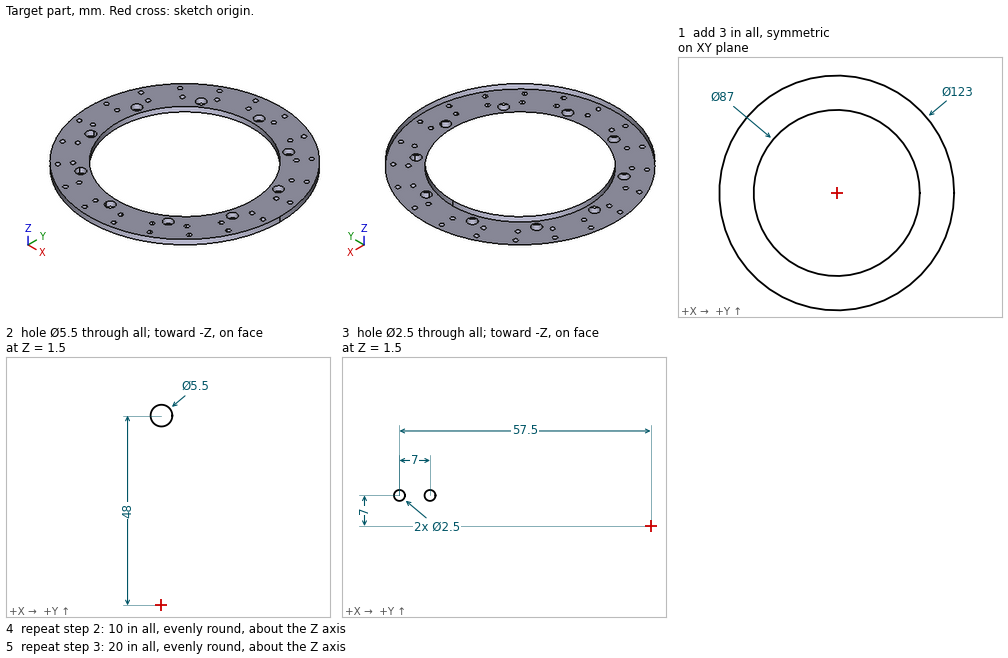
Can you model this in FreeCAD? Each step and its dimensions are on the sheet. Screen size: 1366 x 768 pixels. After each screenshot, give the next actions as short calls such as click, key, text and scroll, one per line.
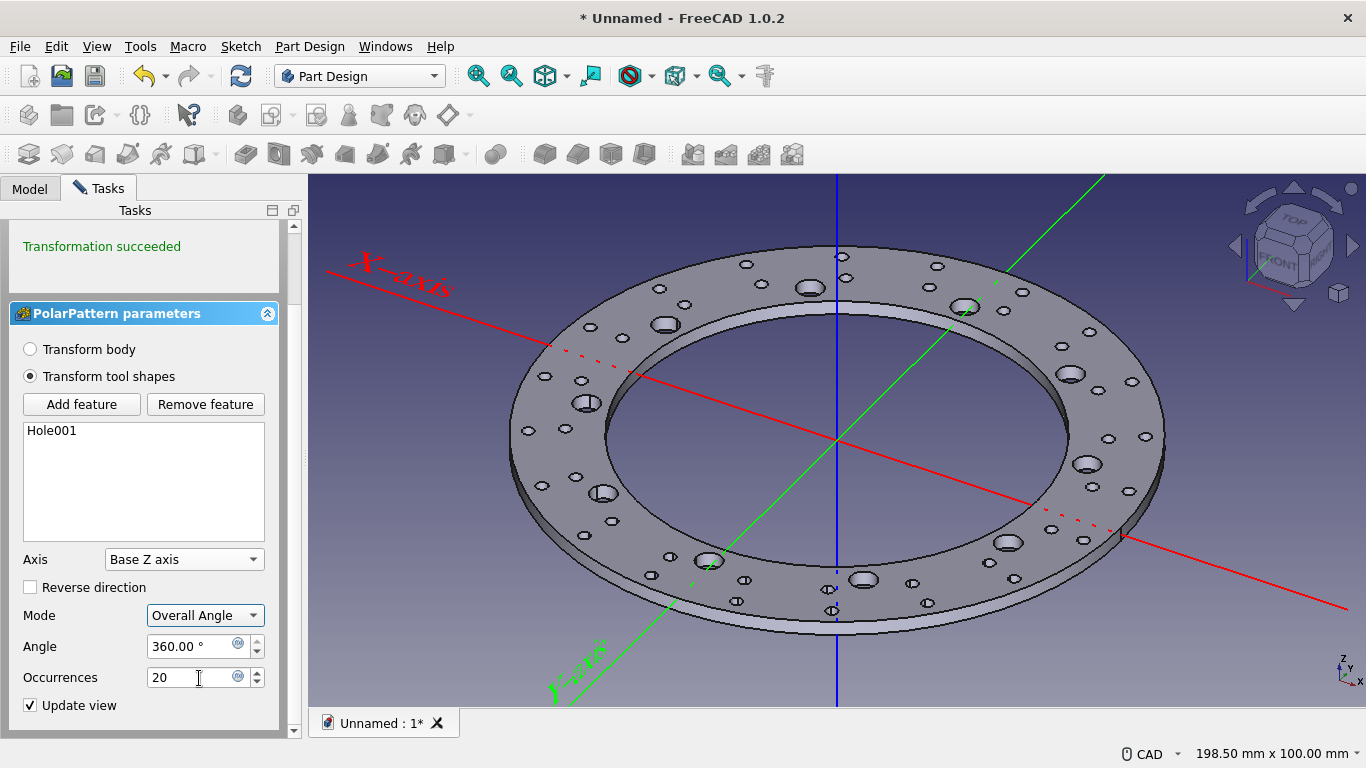
scroll(294, 479, up, 3)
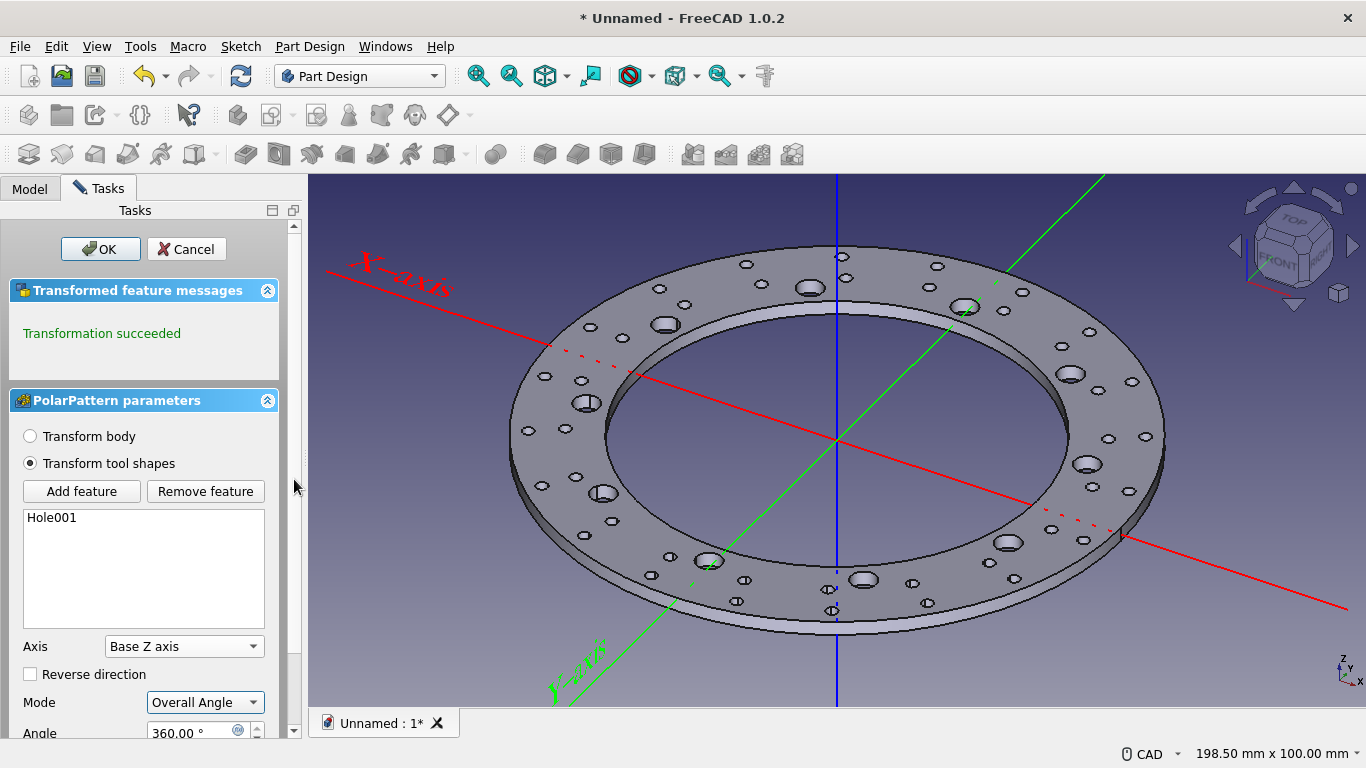
click(101, 249)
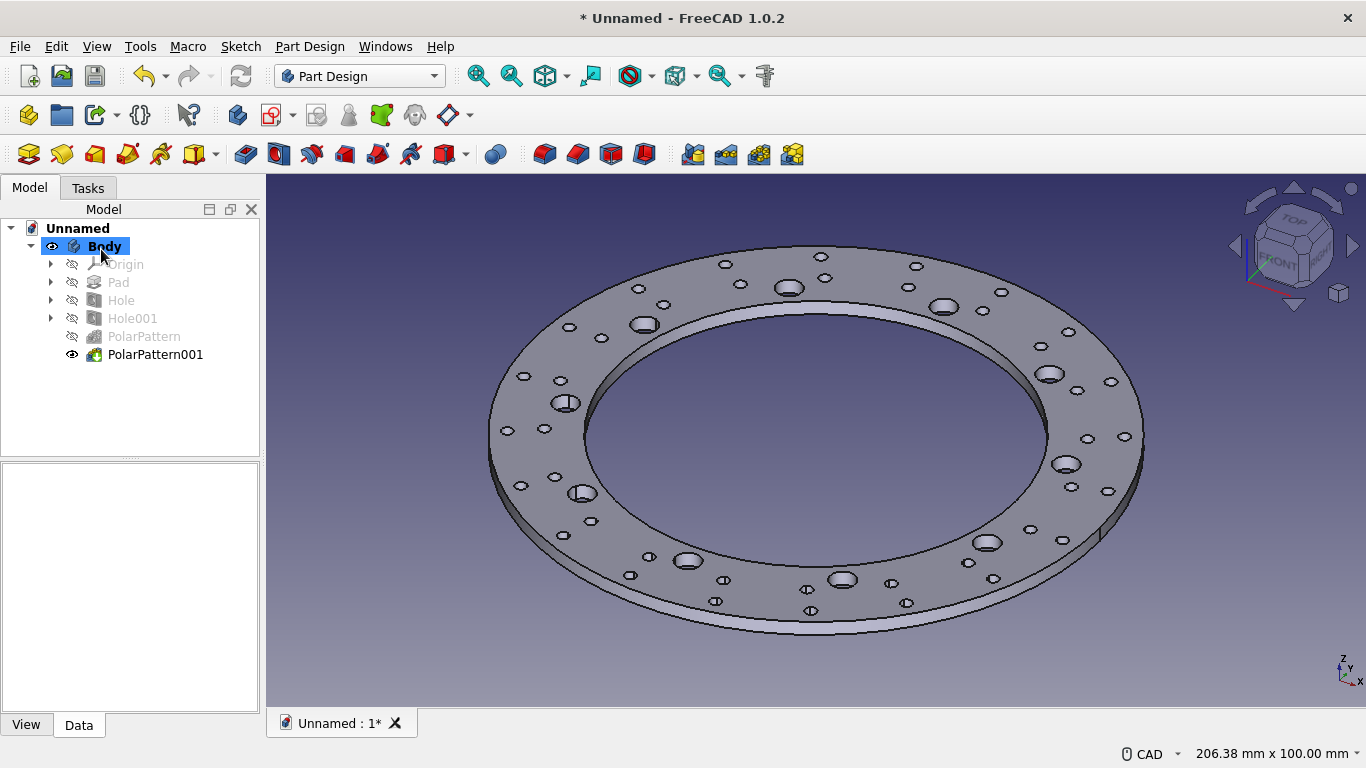
key(0)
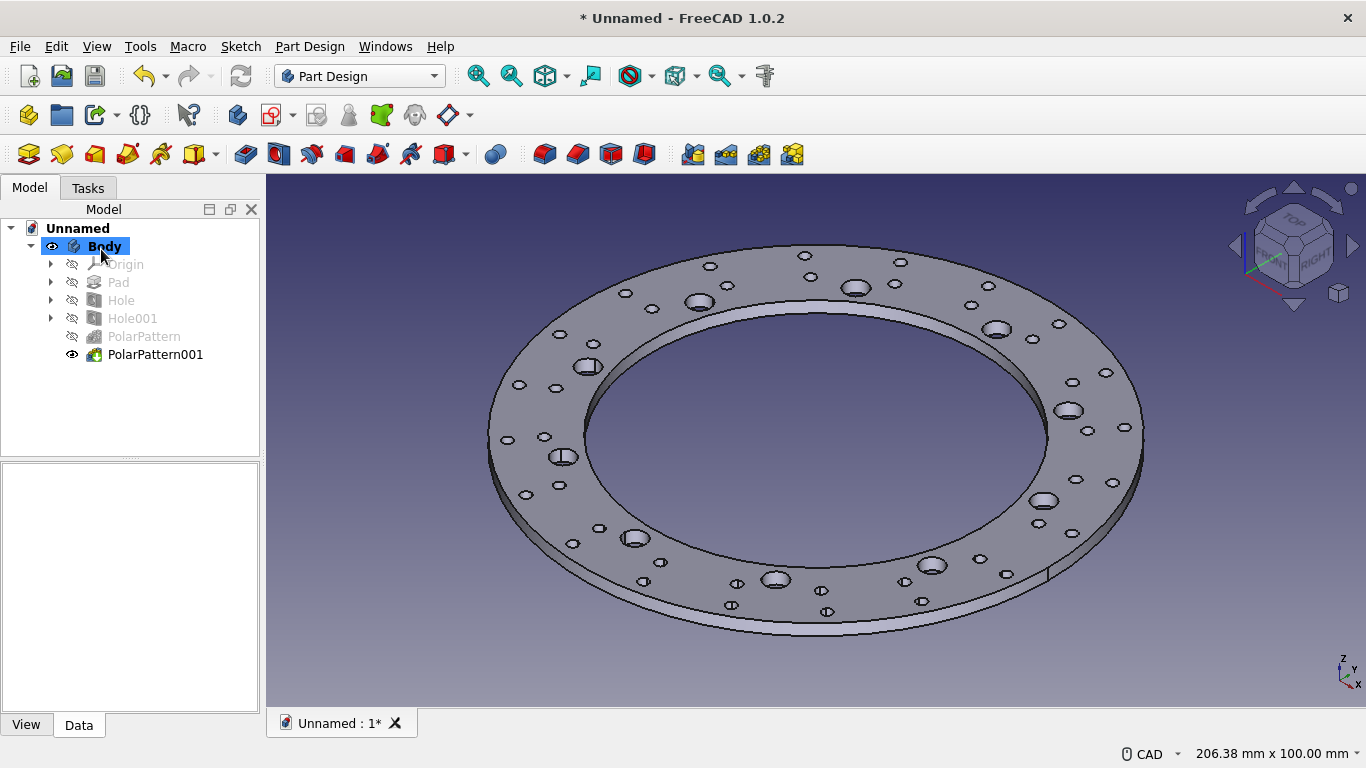
key(v)
key(f)